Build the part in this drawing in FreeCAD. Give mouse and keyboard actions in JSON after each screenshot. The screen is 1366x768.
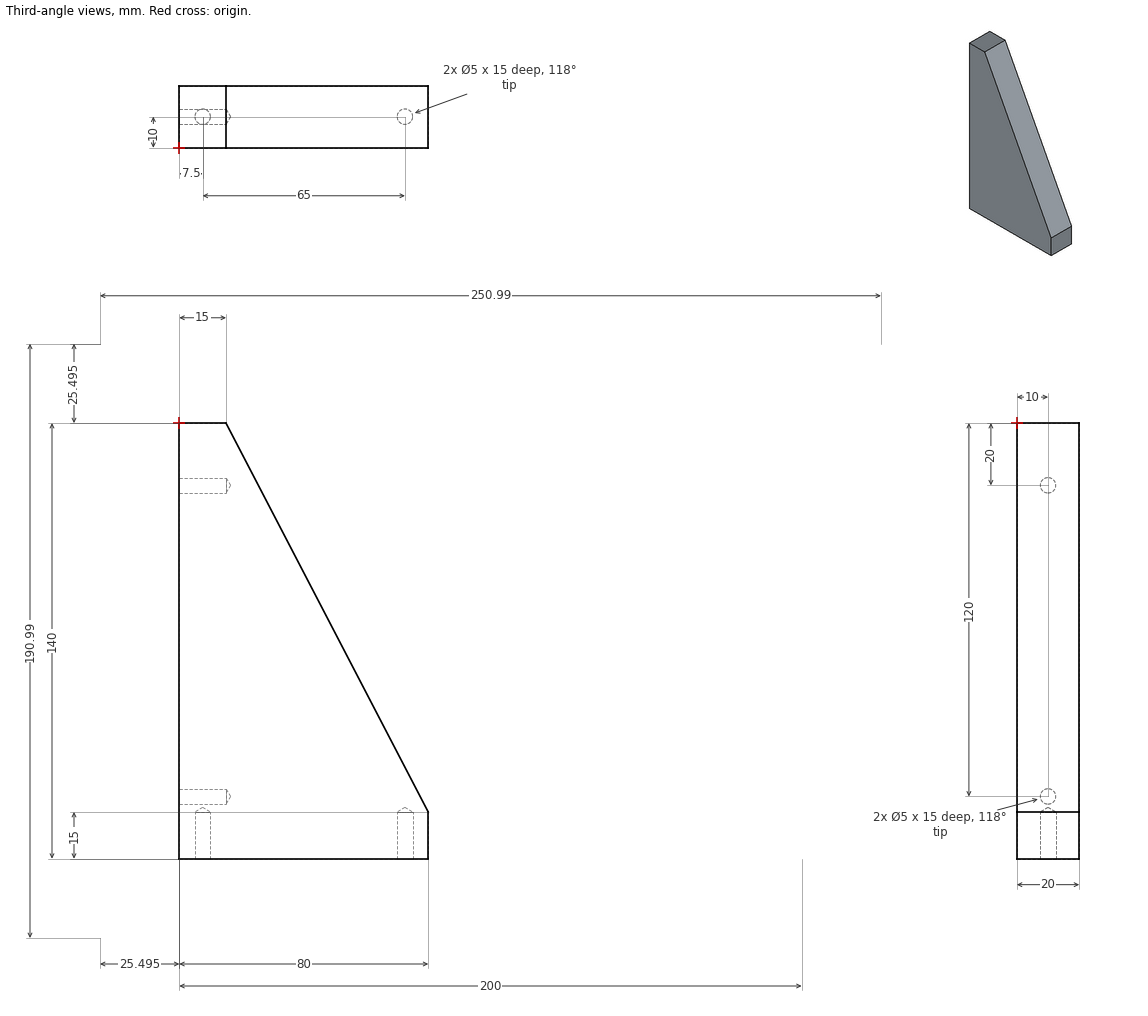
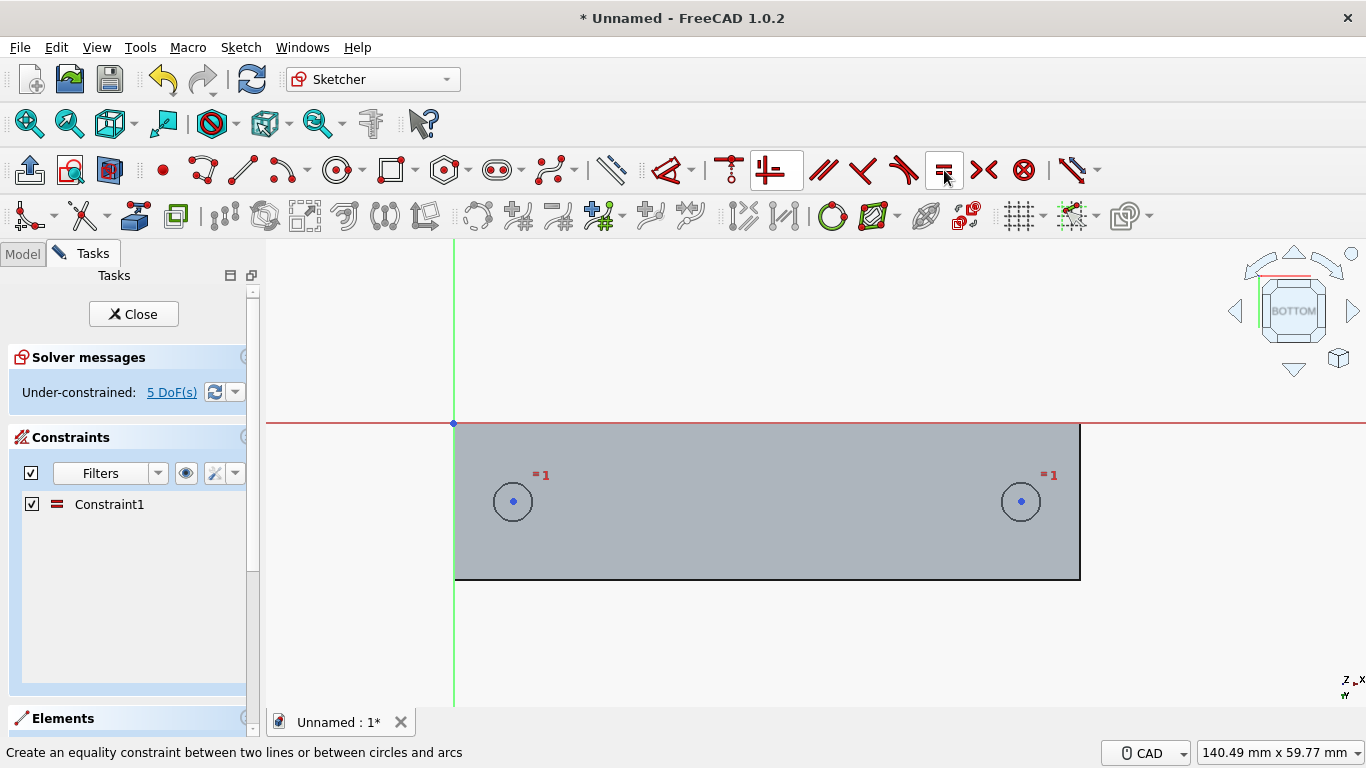
{"action": "key", "text": "d"}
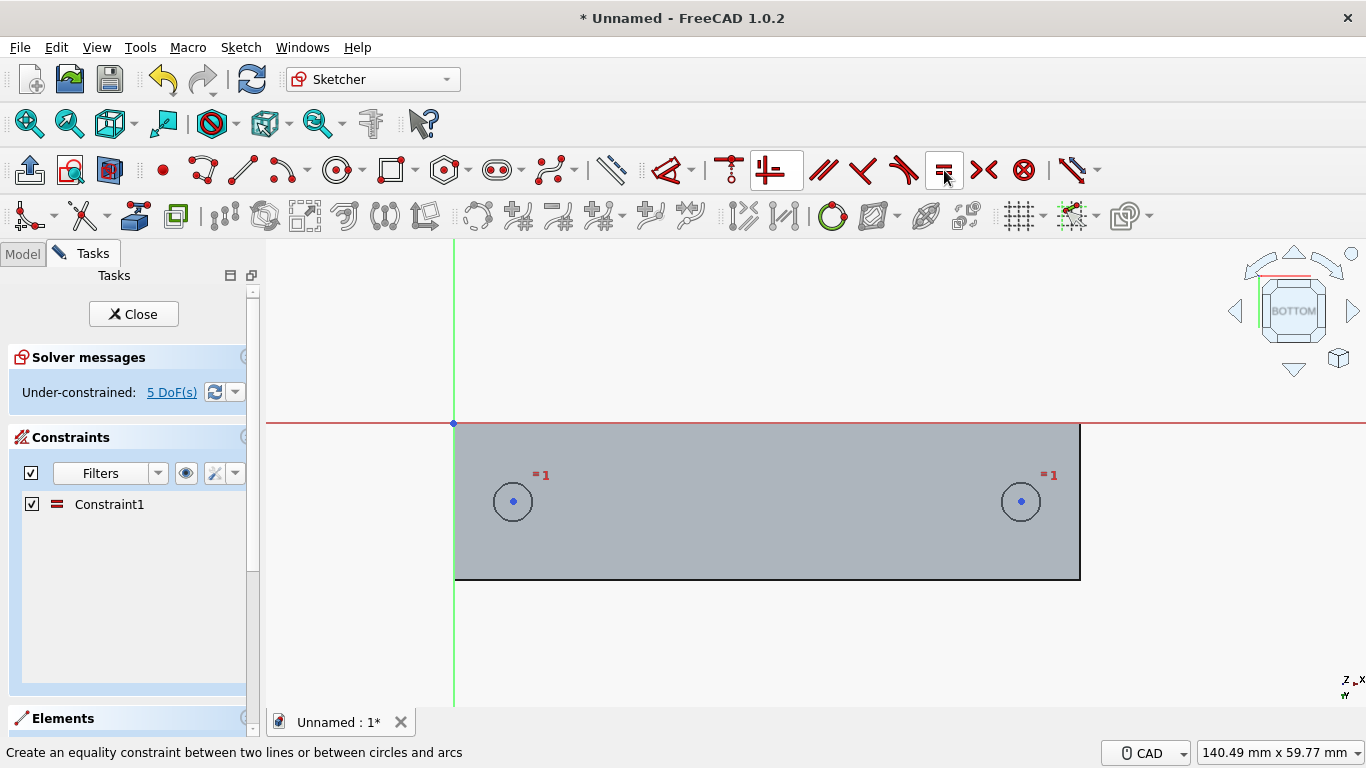
{"action": "left_click", "coordinate": [1034, 488]}
{"action": "left_click", "coordinate": [1056, 465]}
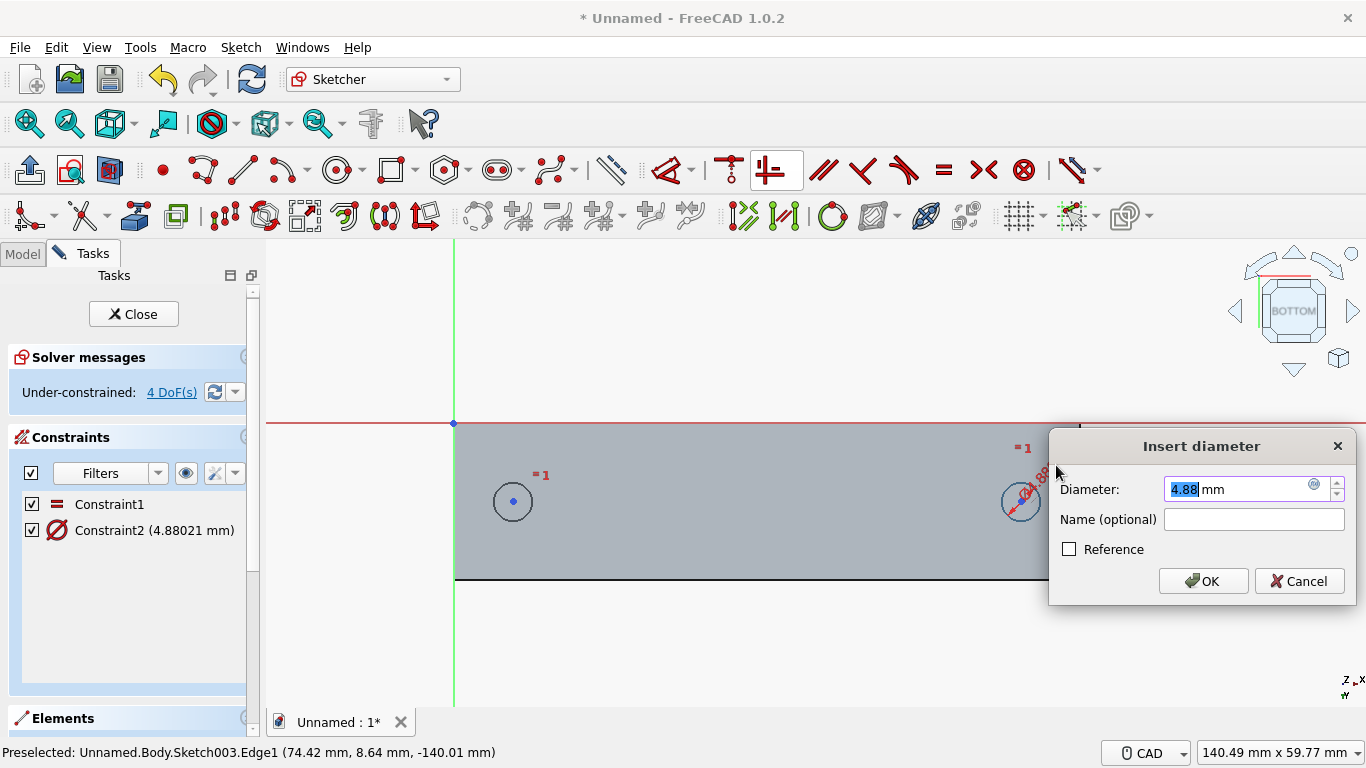
{"action": "type", "text": "5"}
{"action": "key", "text": "Return"}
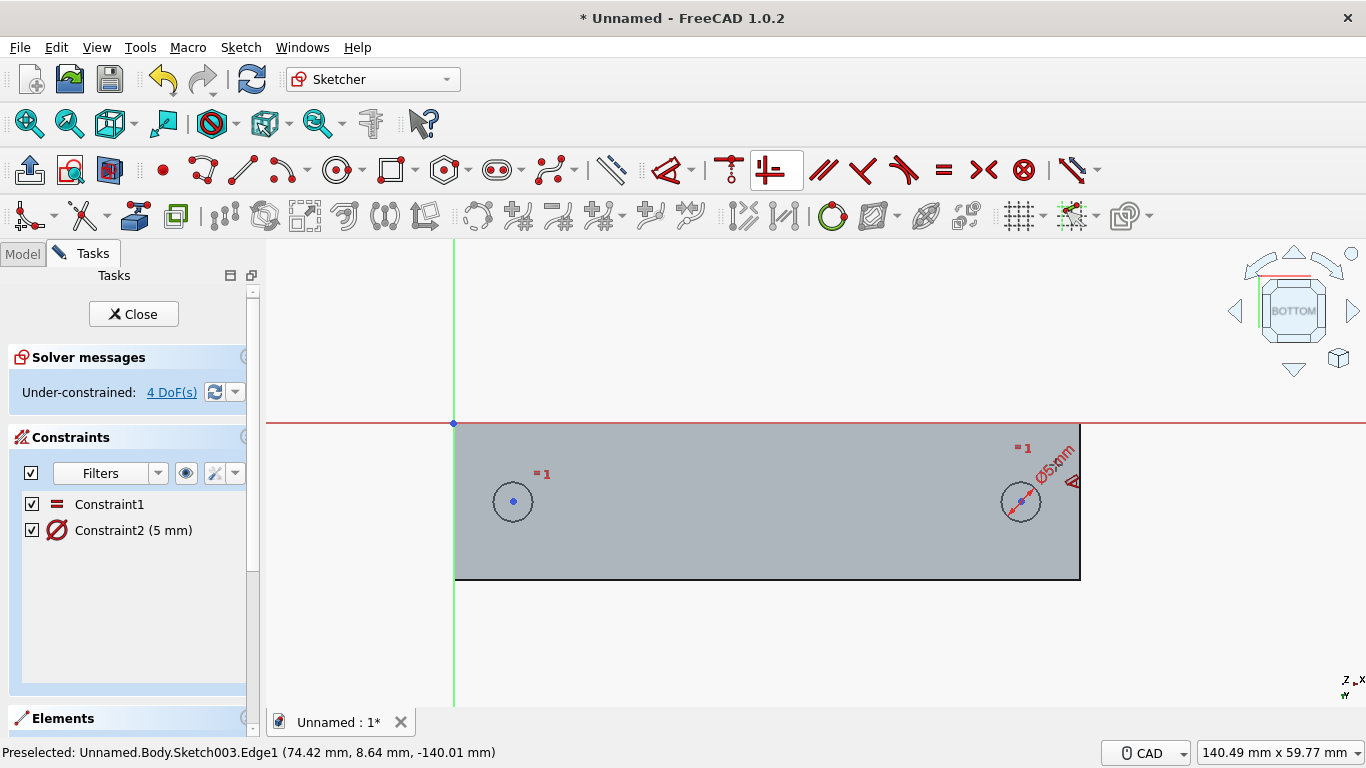
{"action": "left_click", "coordinate": [1021, 502]}
{"action": "left_click", "coordinate": [420, 463]}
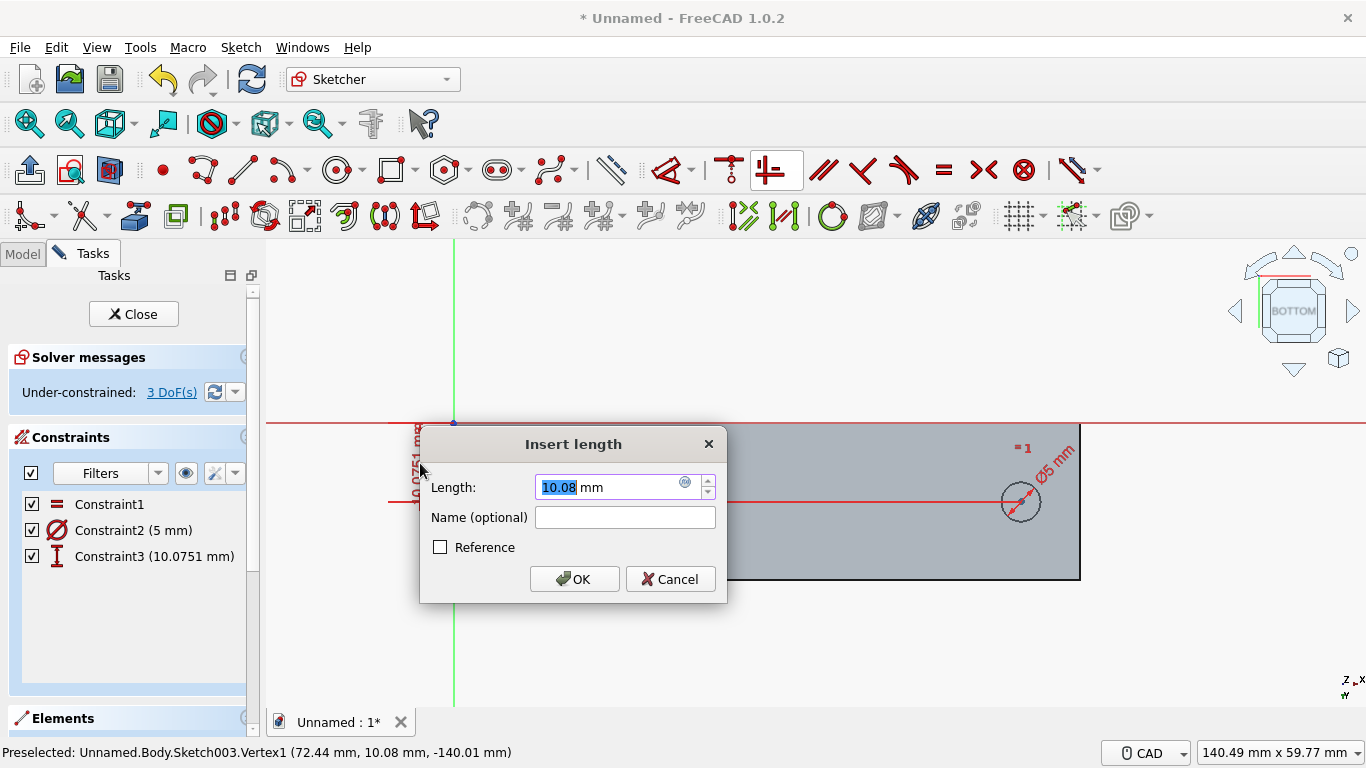
{"action": "type", "text": "10"}
{"action": "key", "text": "Return"}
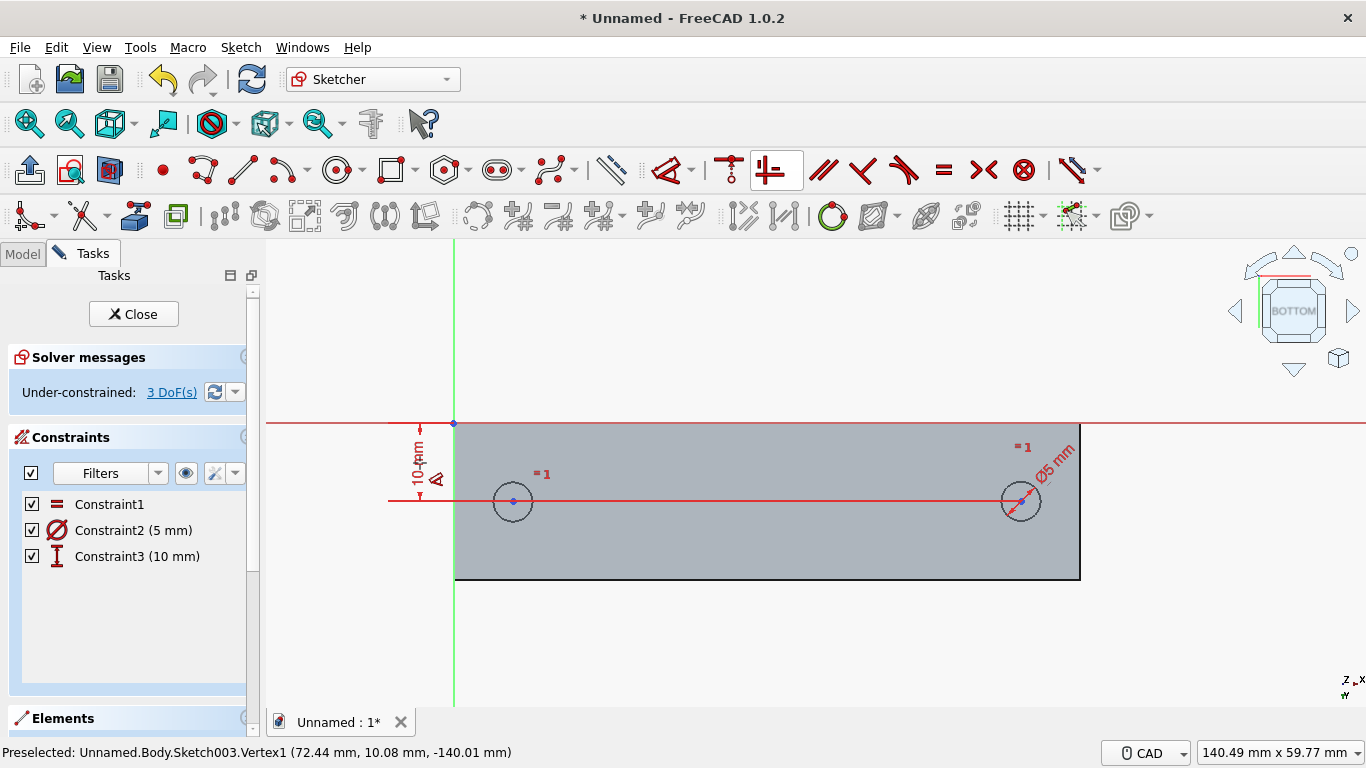
{"action": "left_click", "coordinate": [513, 502]}
{"action": "left_click", "coordinate": [420, 490]}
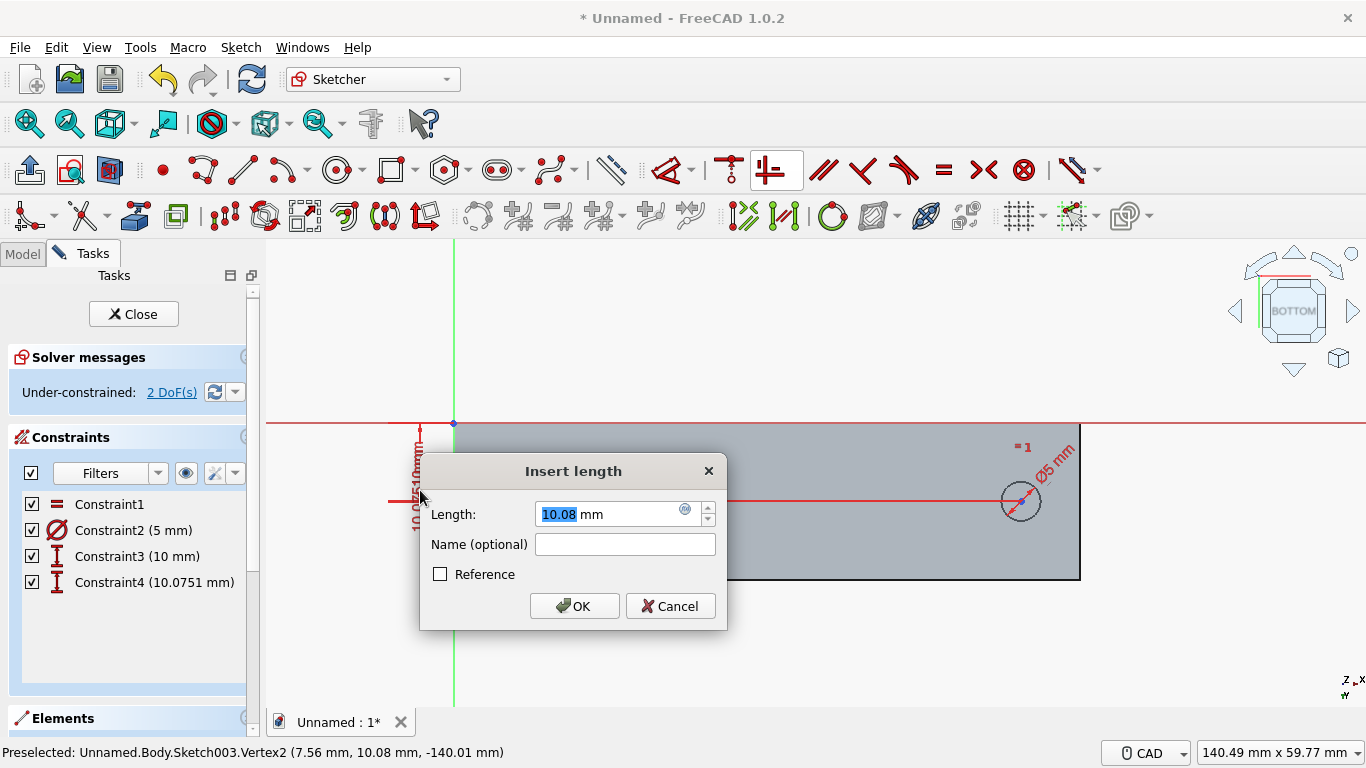
{"action": "type", "text": "10"}
{"action": "key", "text": "Return"}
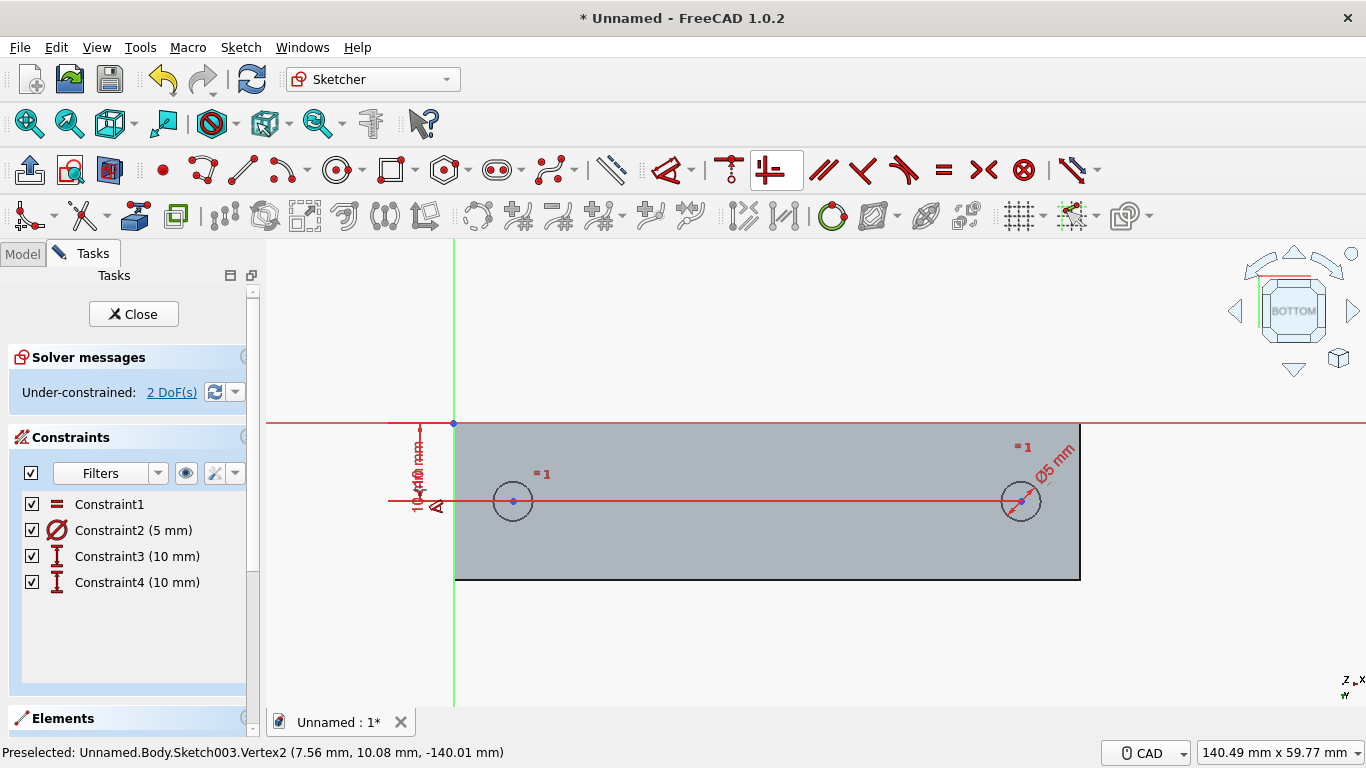
{"action": "left_click", "coordinate": [513, 501]}
{"action": "left_click", "coordinate": [483, 389]}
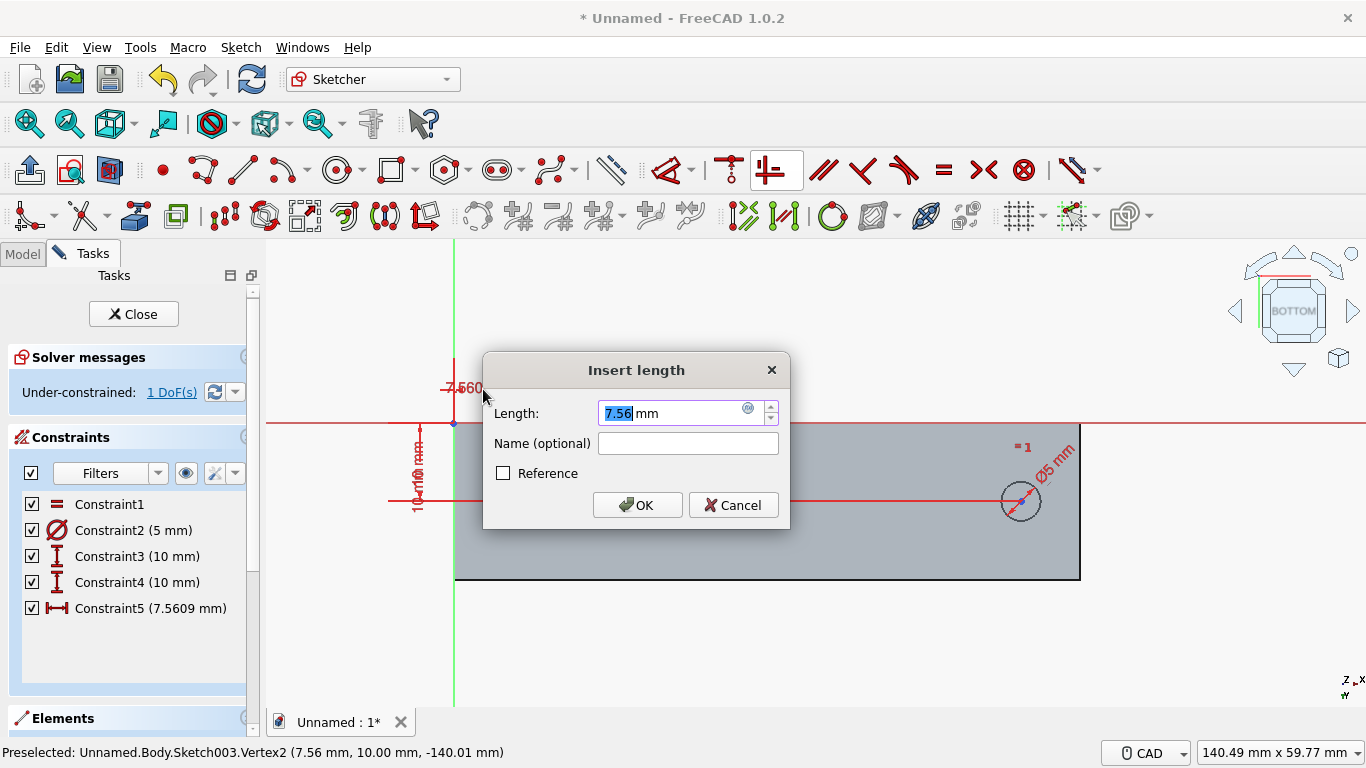
{"action": "type", "text": "7.5"}
{"action": "key", "text": "Return"}